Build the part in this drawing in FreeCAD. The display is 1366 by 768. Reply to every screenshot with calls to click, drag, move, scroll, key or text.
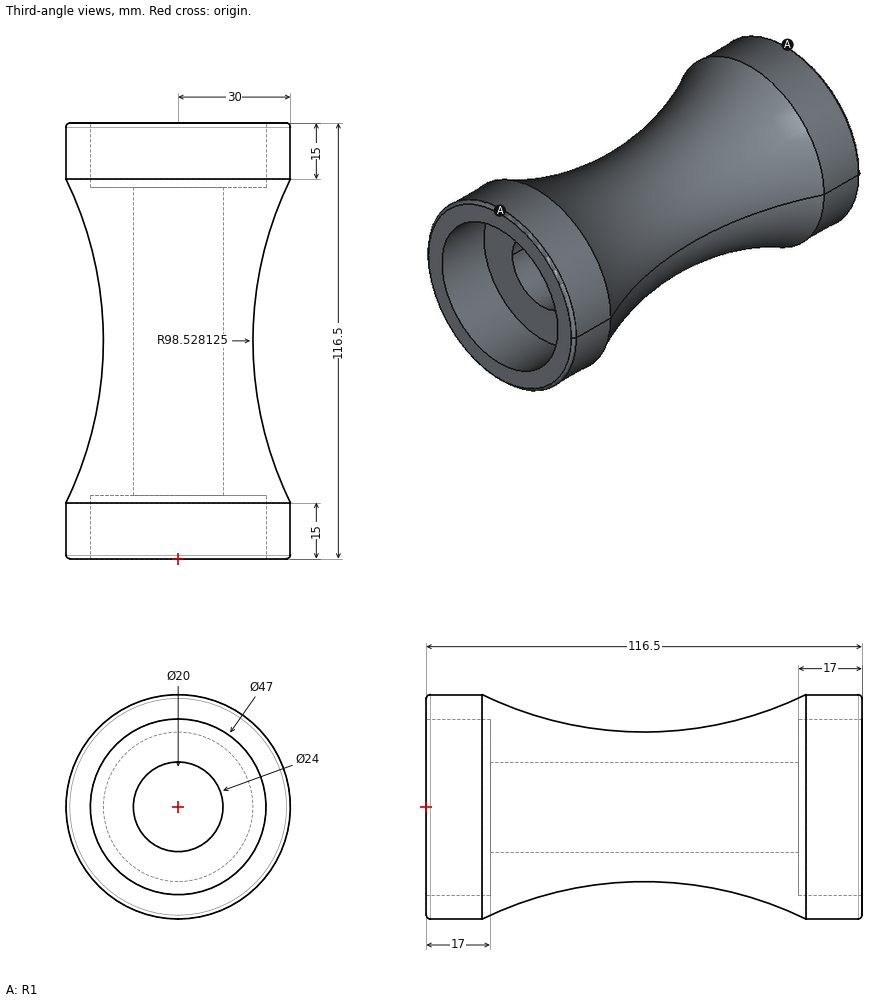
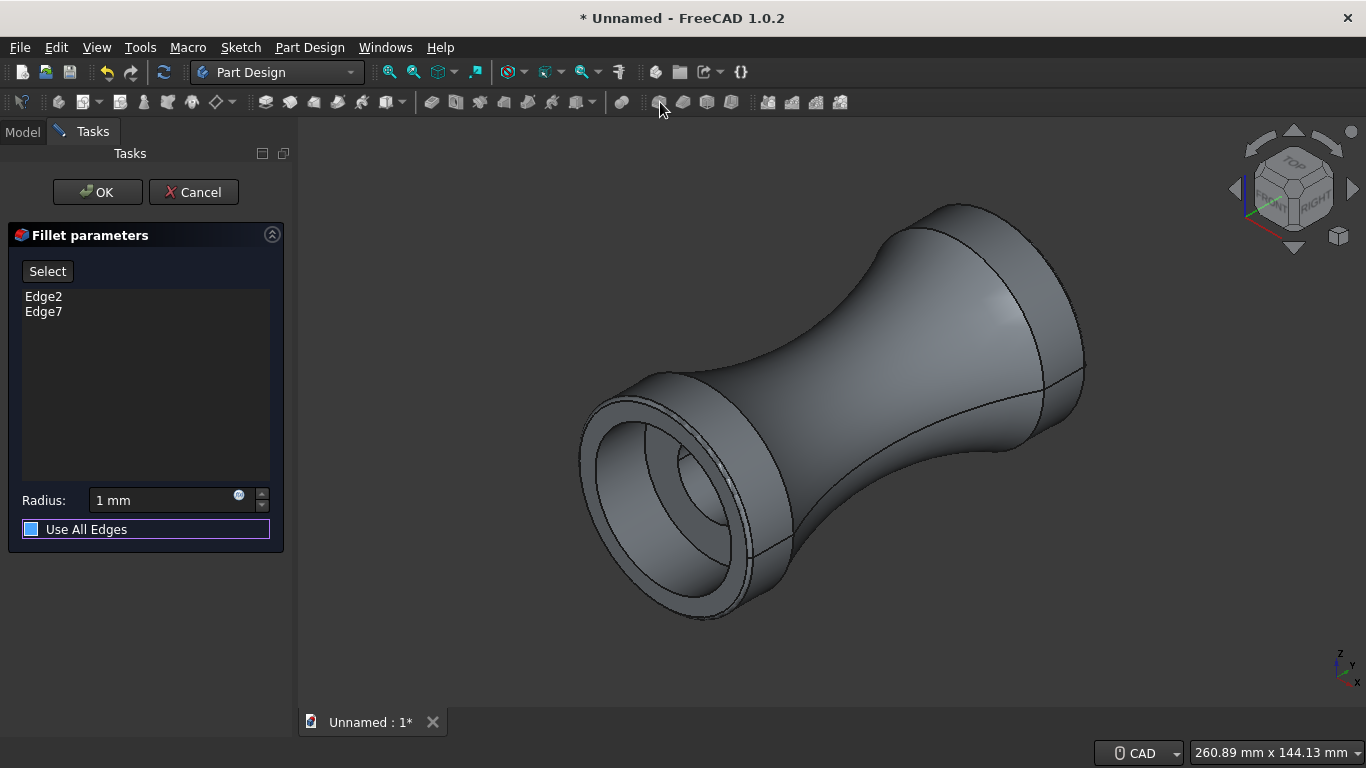
click(98, 192)